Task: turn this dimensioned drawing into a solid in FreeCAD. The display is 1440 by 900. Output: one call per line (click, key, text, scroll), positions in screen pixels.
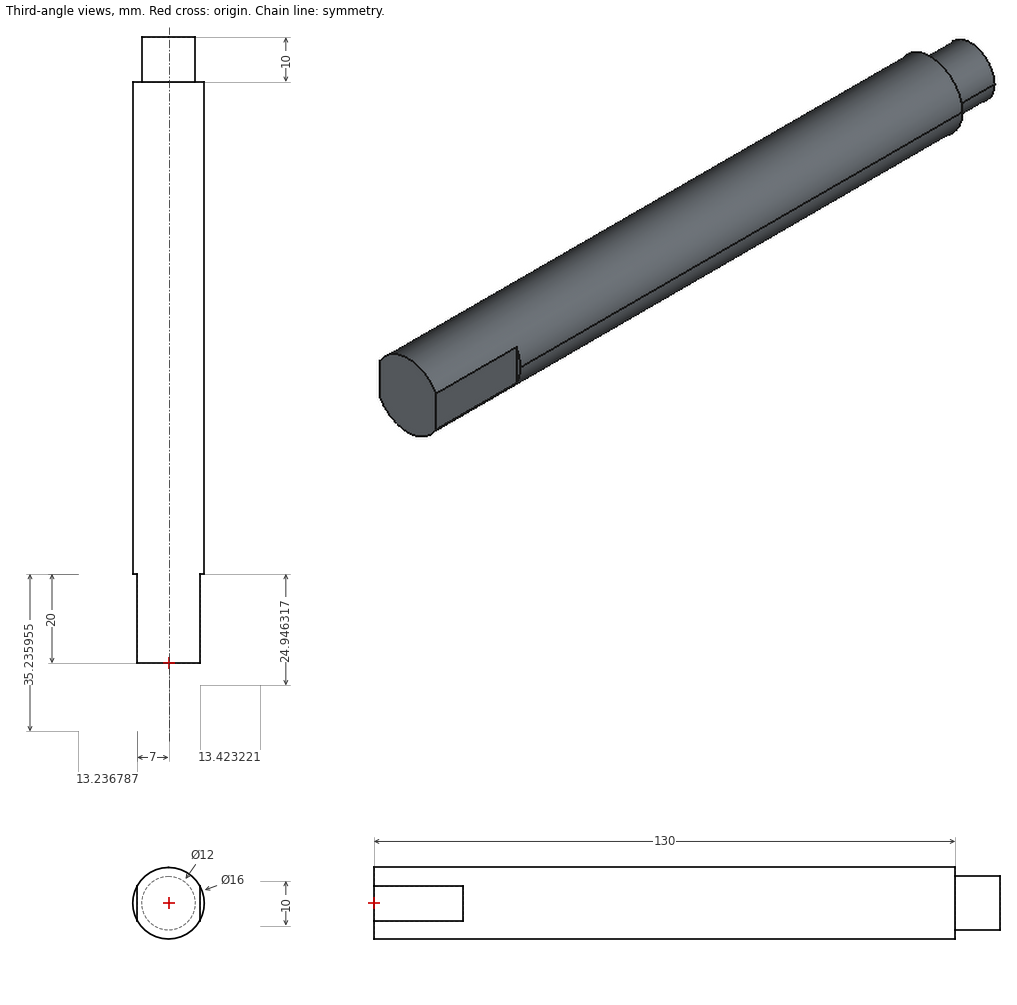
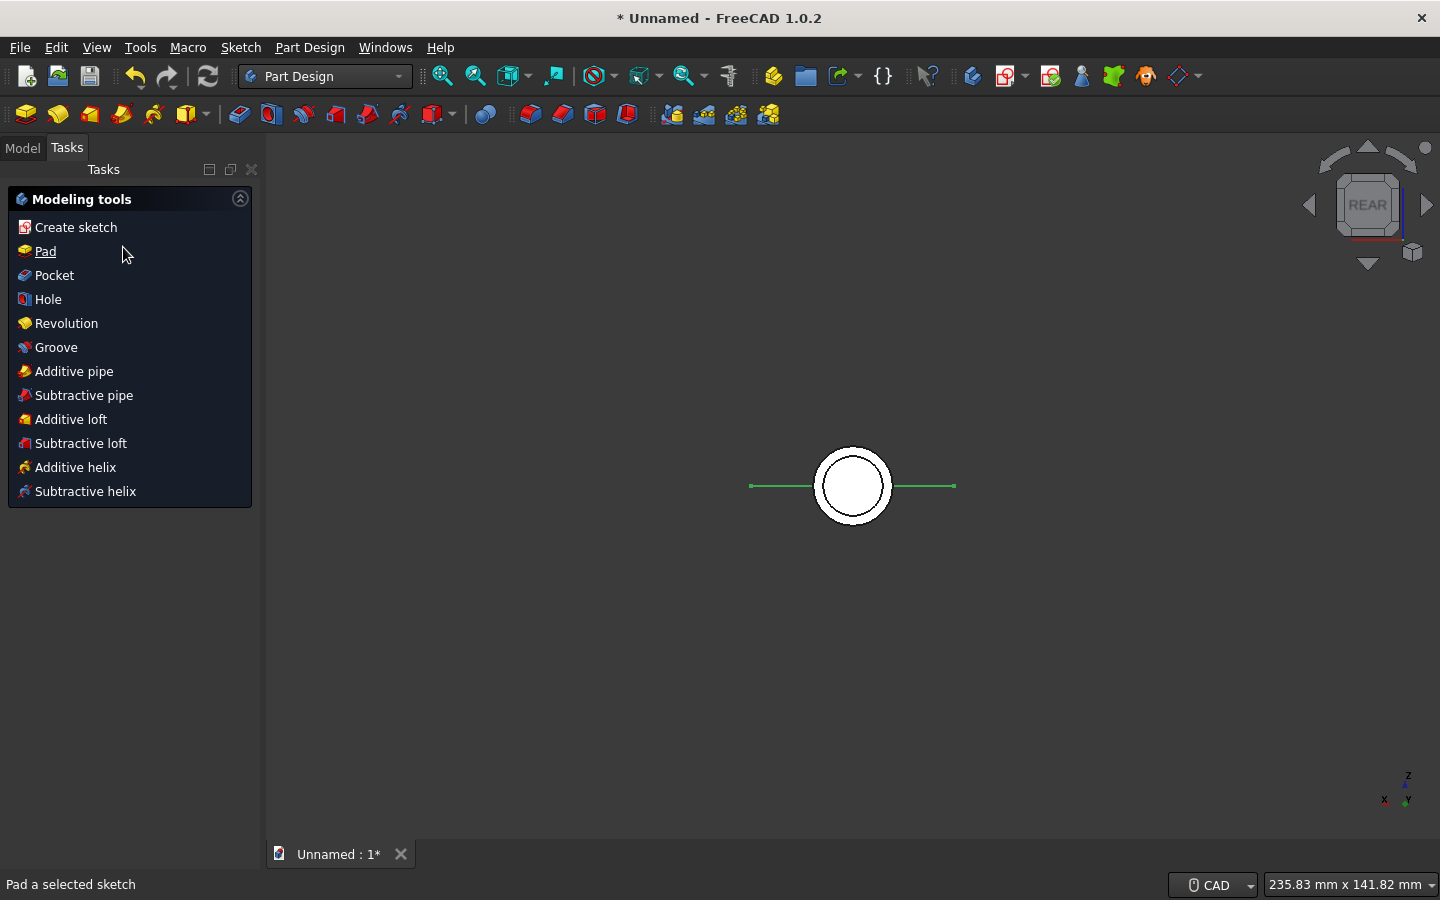
click(240, 114)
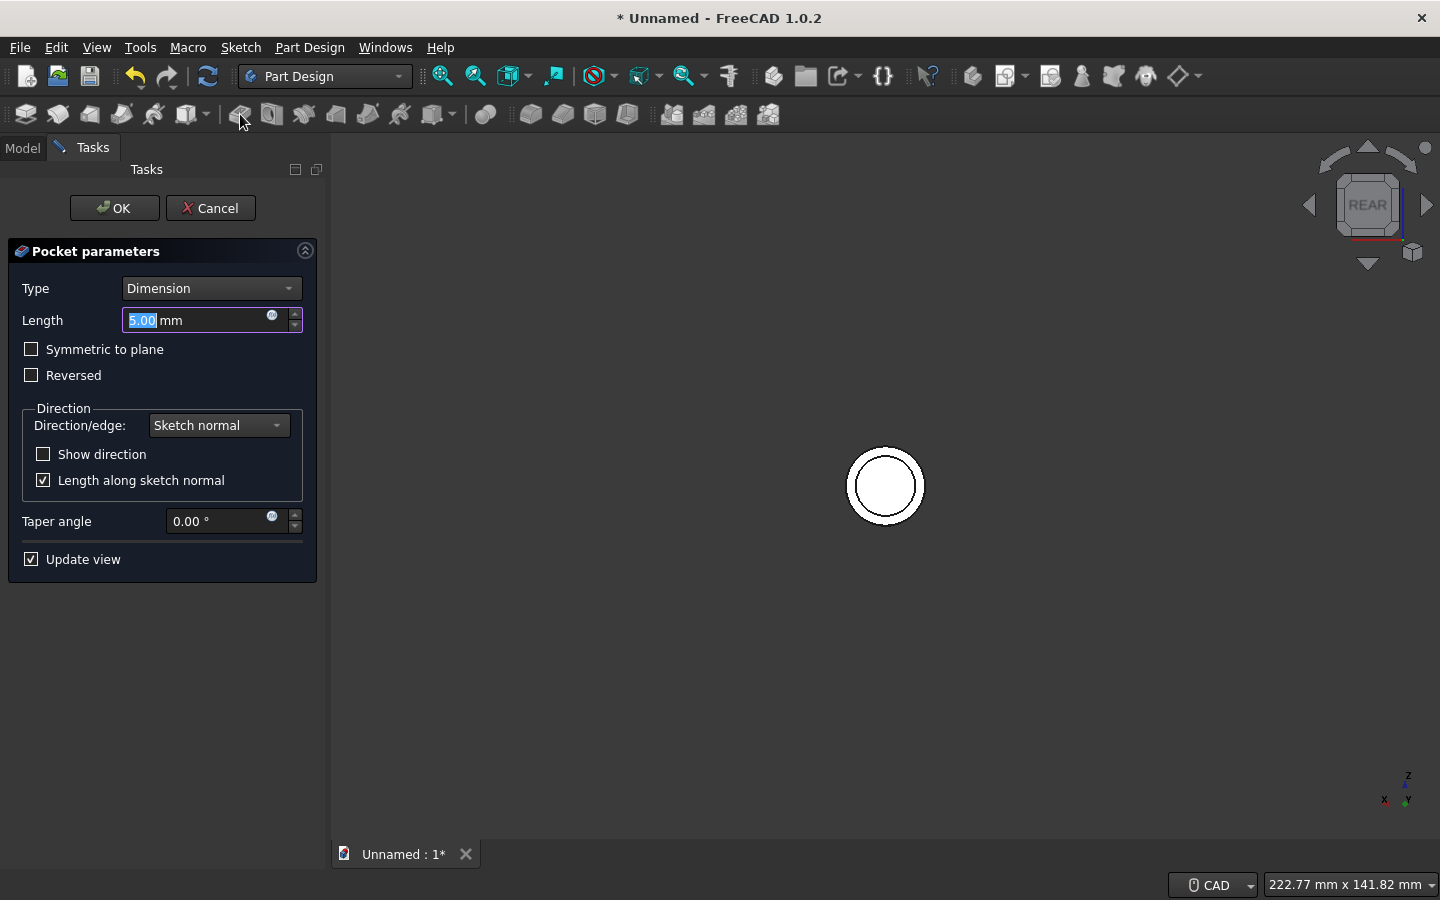
text(10)
key(Tab)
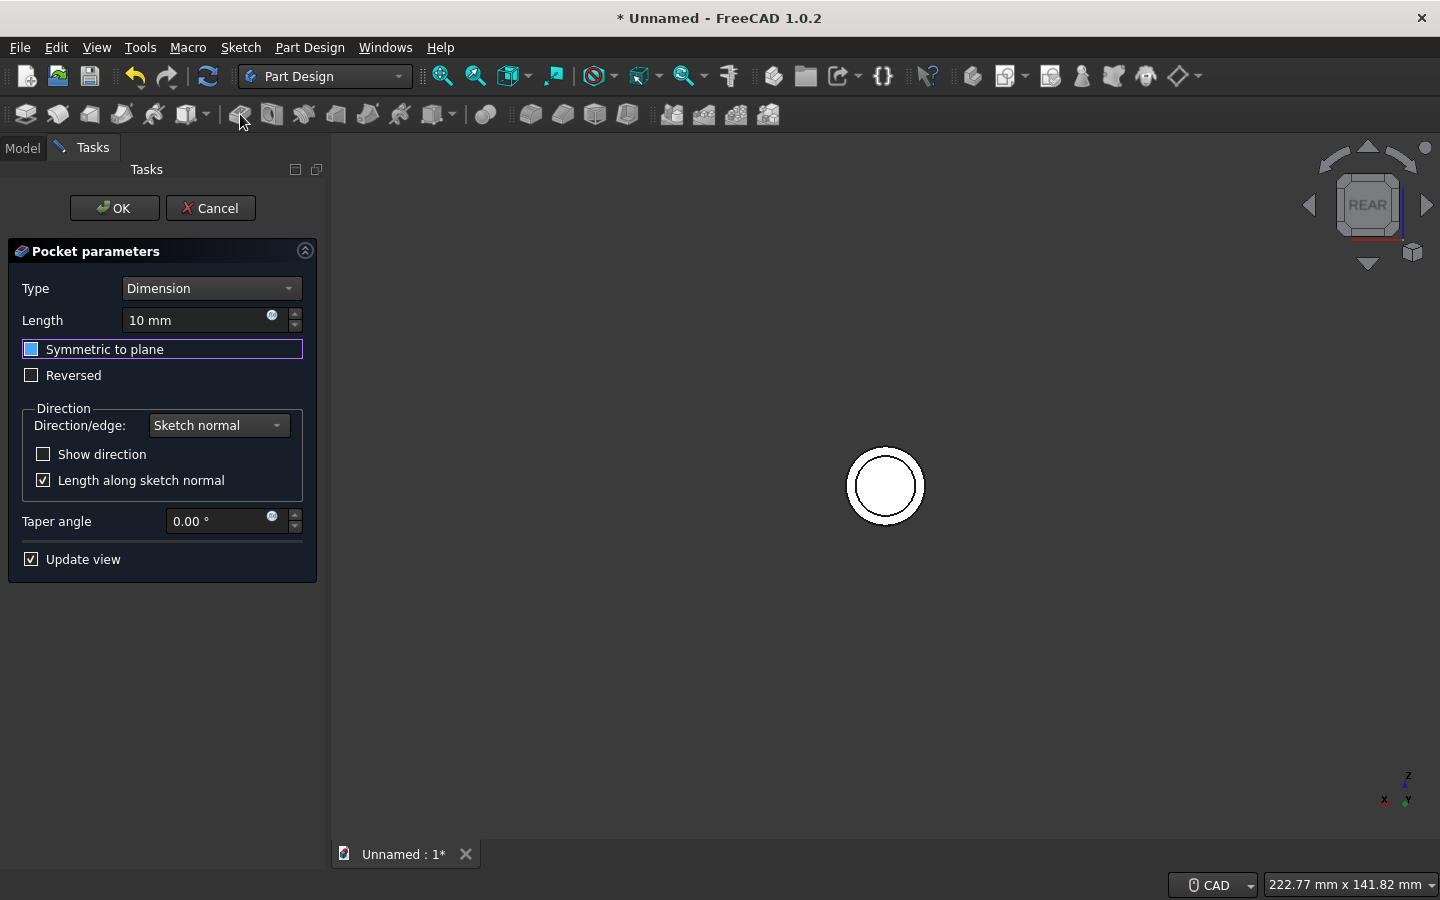
click(30, 349)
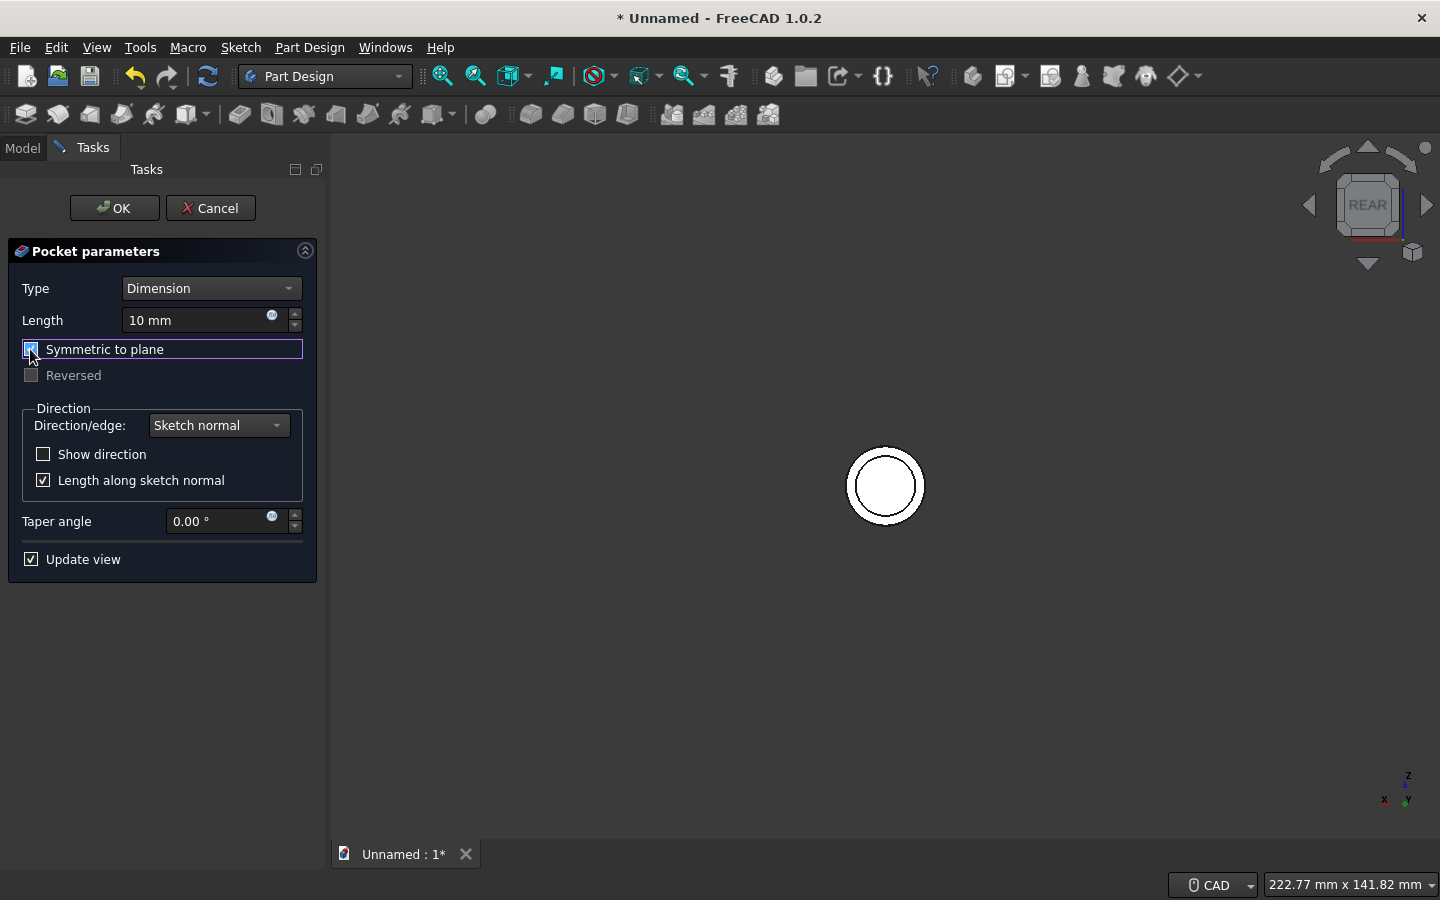
click(115, 208)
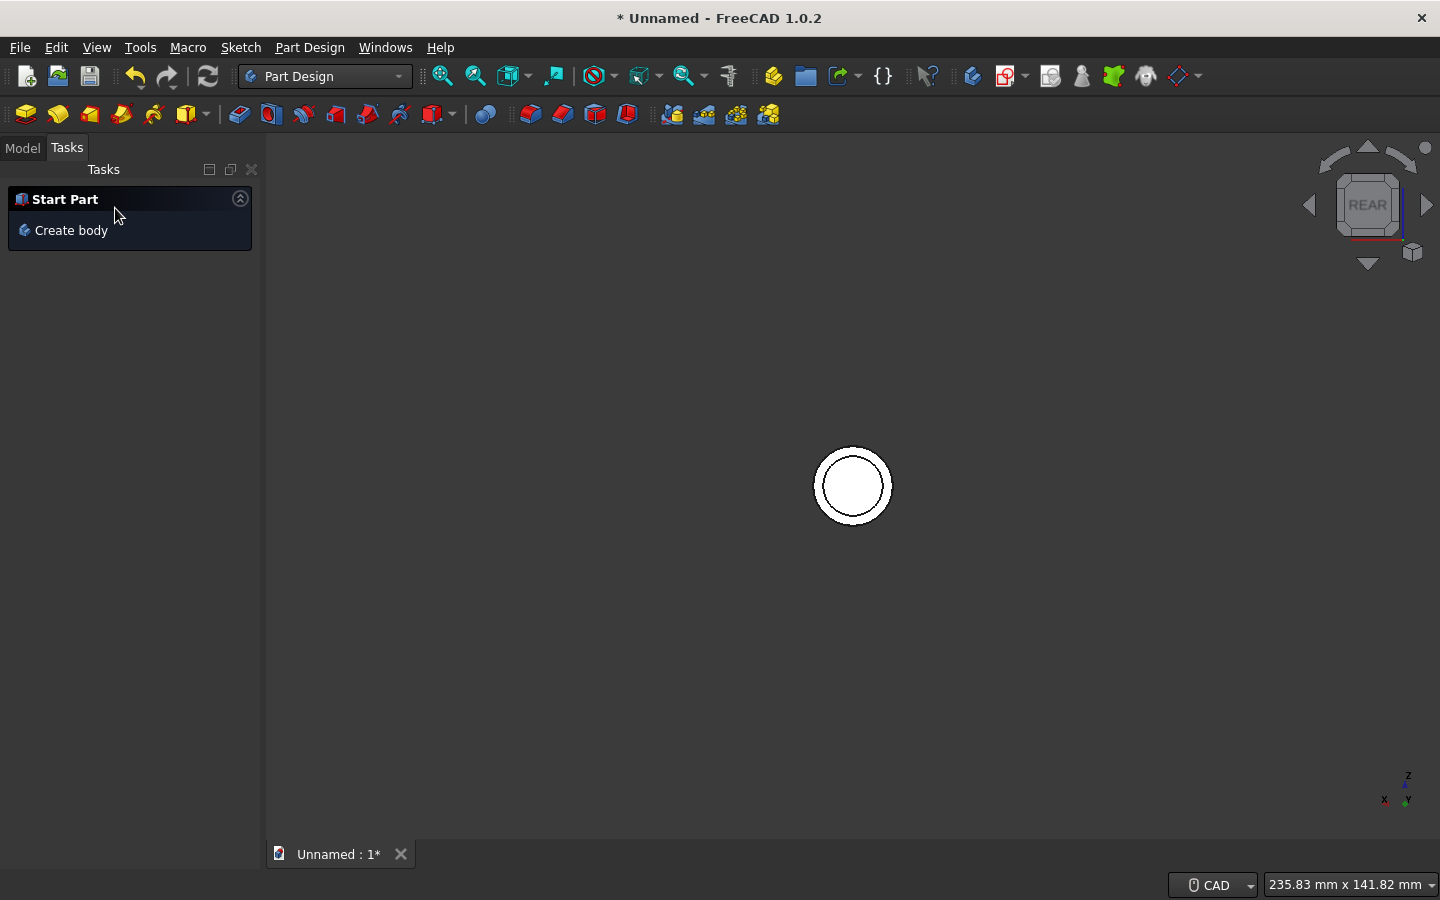
key(0)